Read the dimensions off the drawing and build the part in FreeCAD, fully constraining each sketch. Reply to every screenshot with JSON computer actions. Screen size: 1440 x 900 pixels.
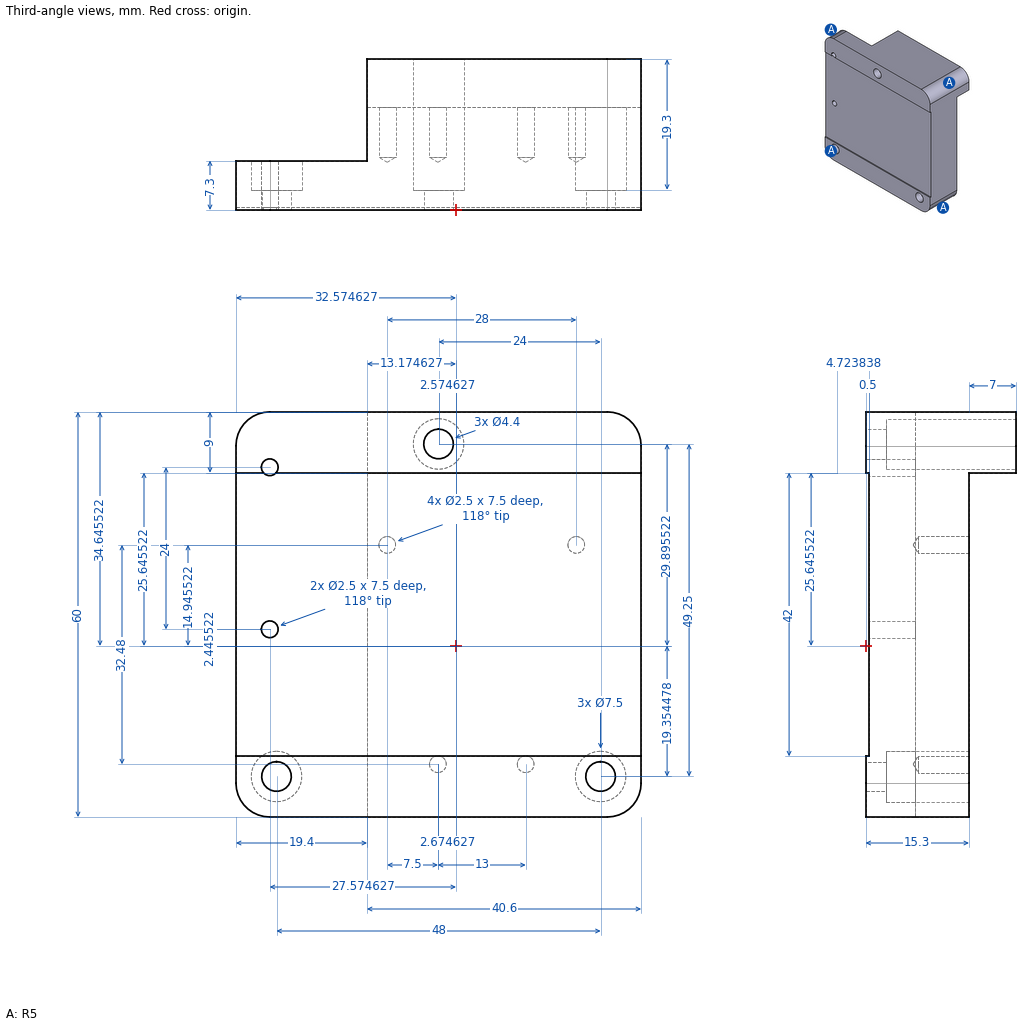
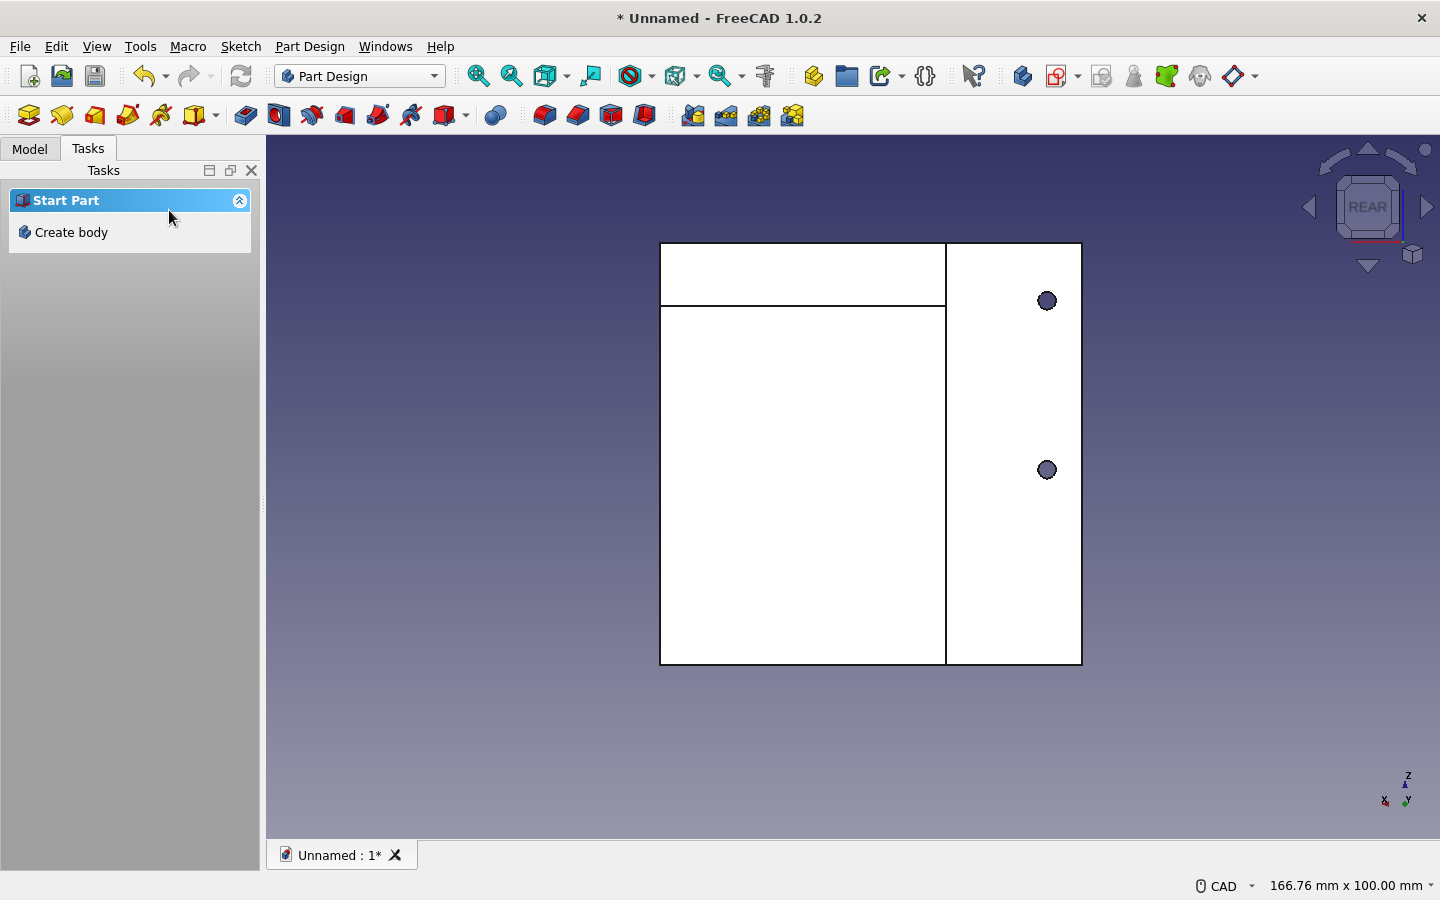
{"action": "left_click", "coordinate": [803, 485]}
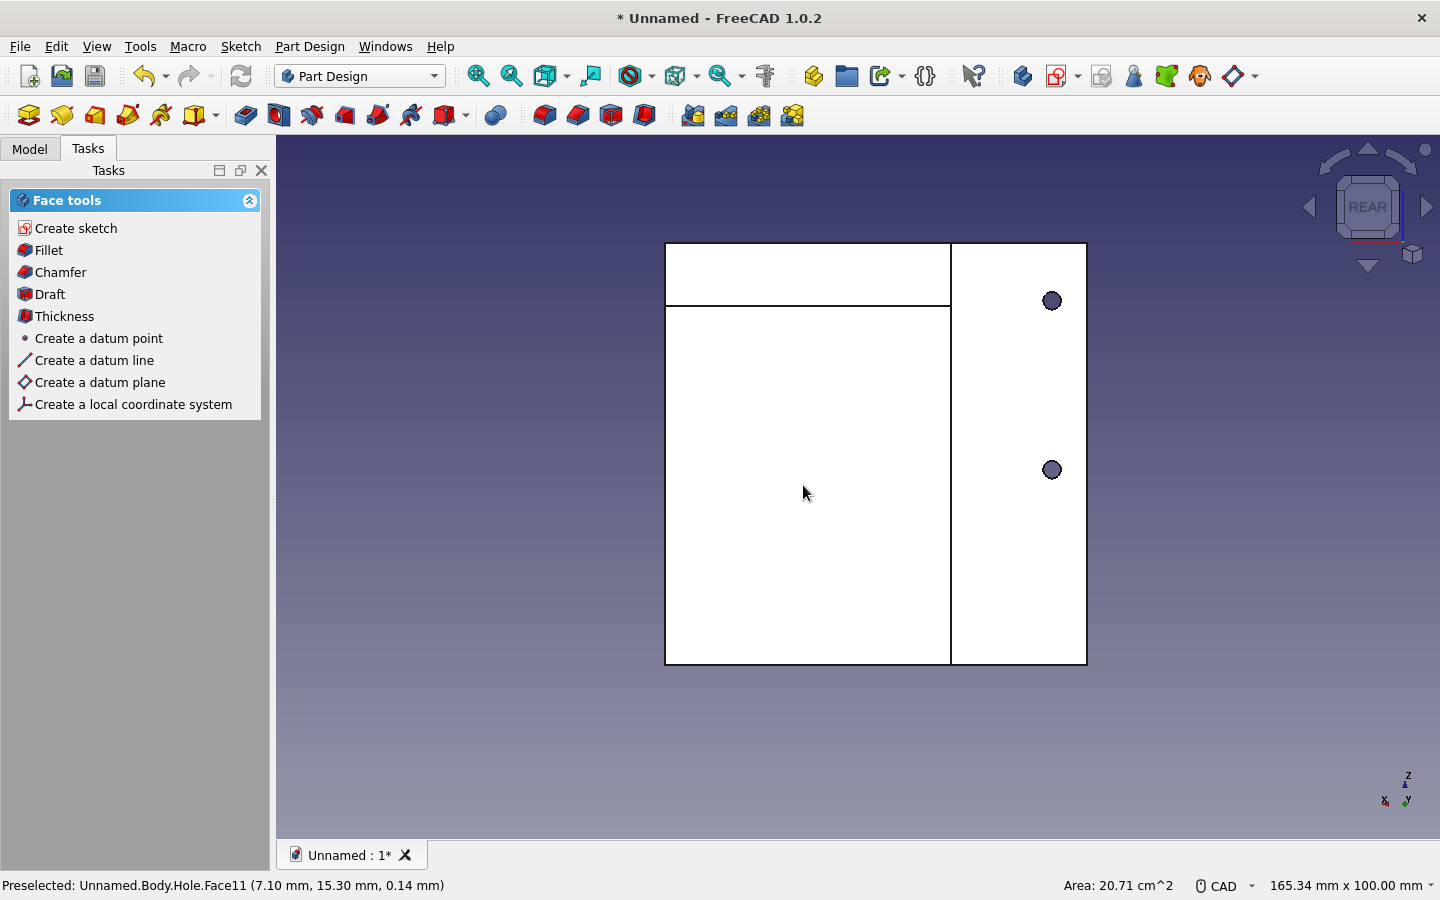
{"action": "left_click", "coordinate": [1056, 76]}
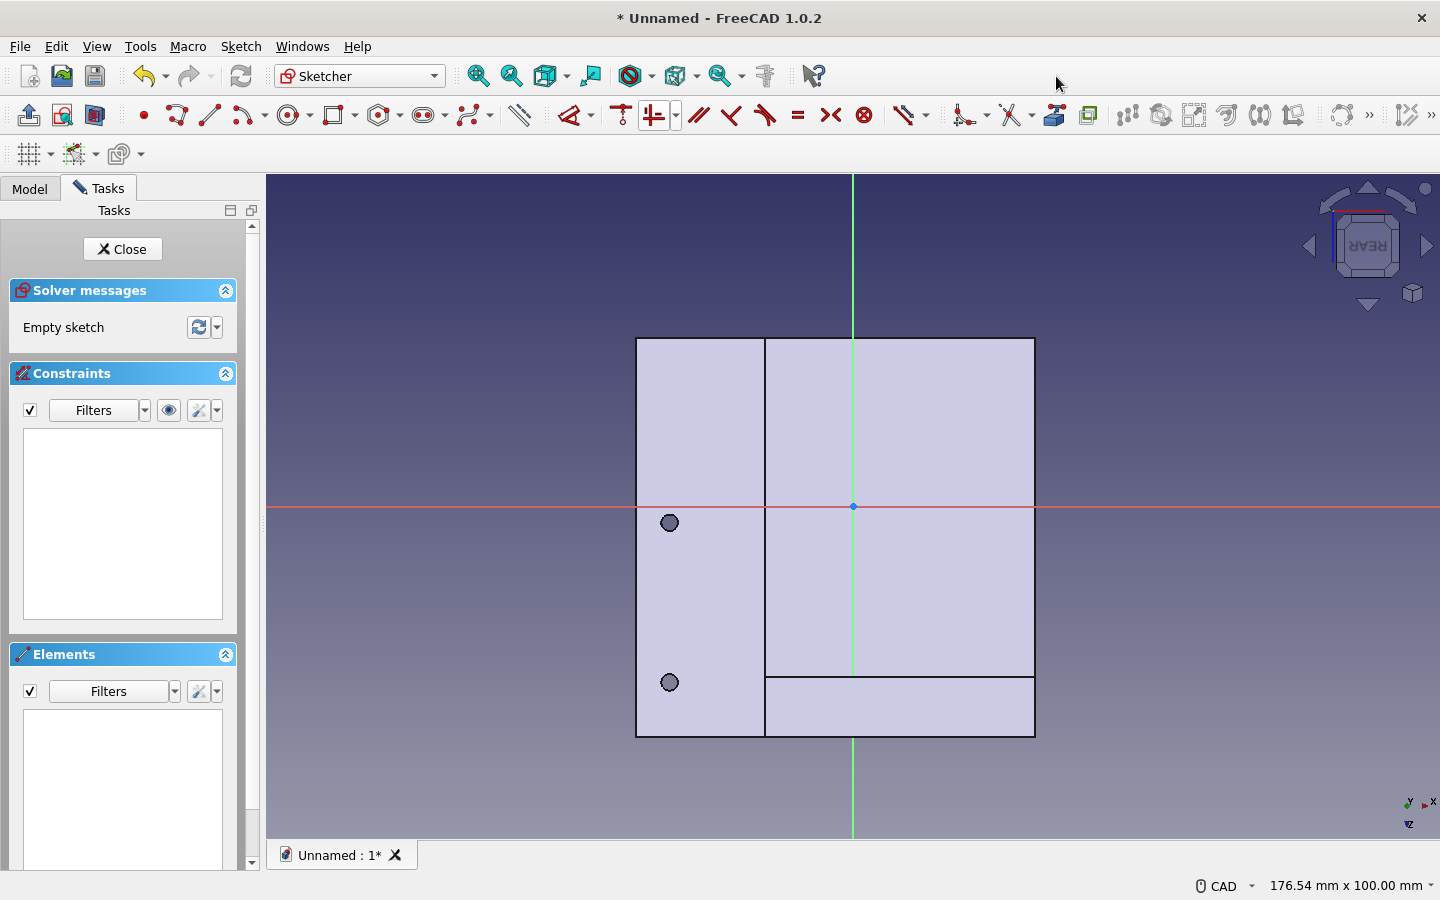
{"action": "scroll", "coordinate": [993, 487], "scroll_direction": "up", "scroll_amount": 3}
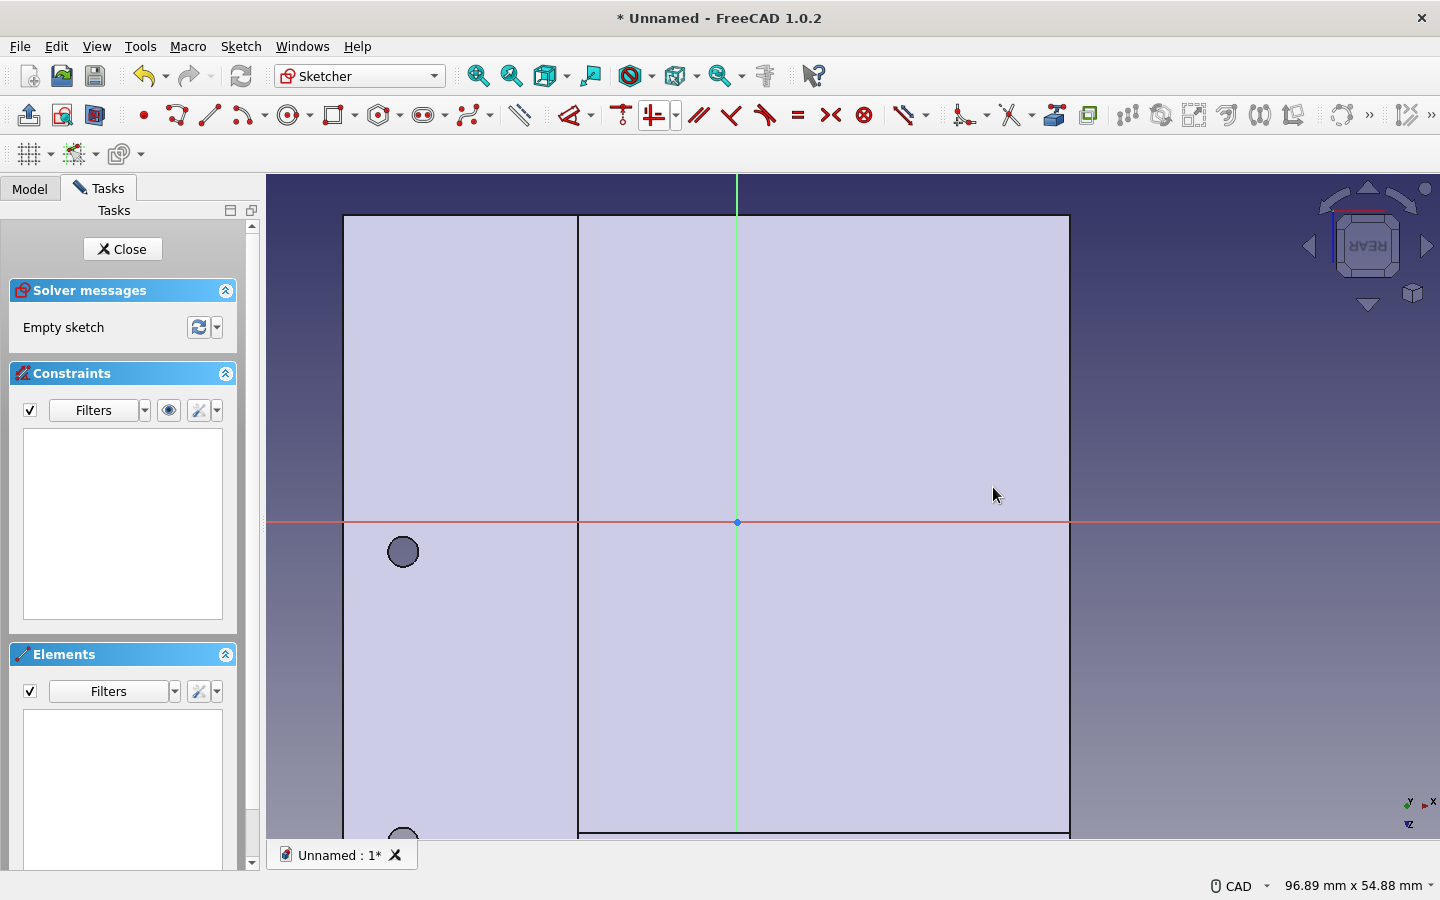
{"action": "key", "text": "g c"}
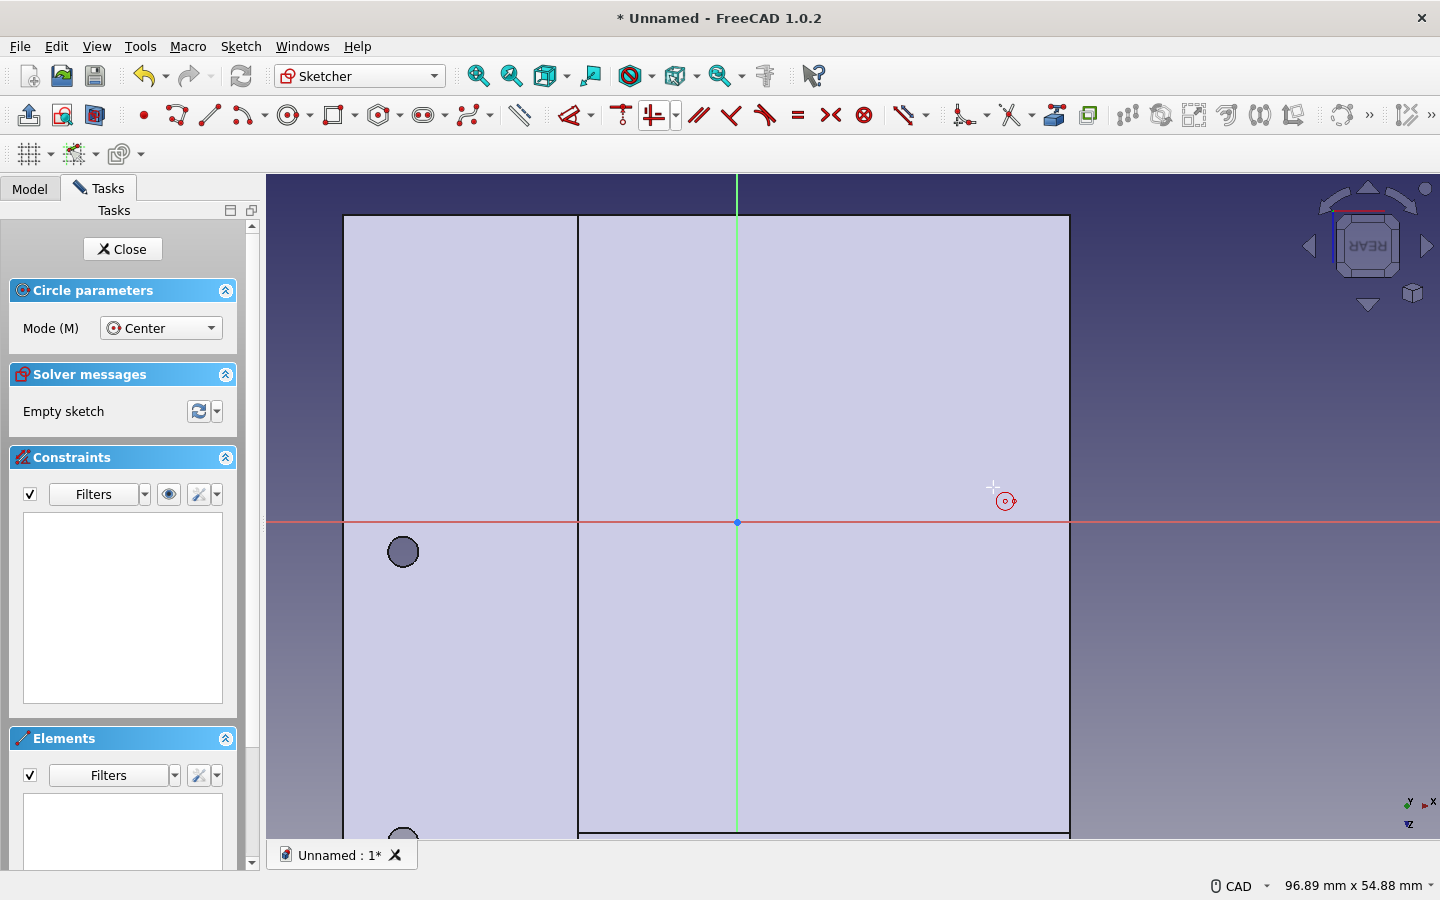
{"action": "scroll", "coordinate": [614, 703], "scroll_direction": "up", "scroll_amount": 3}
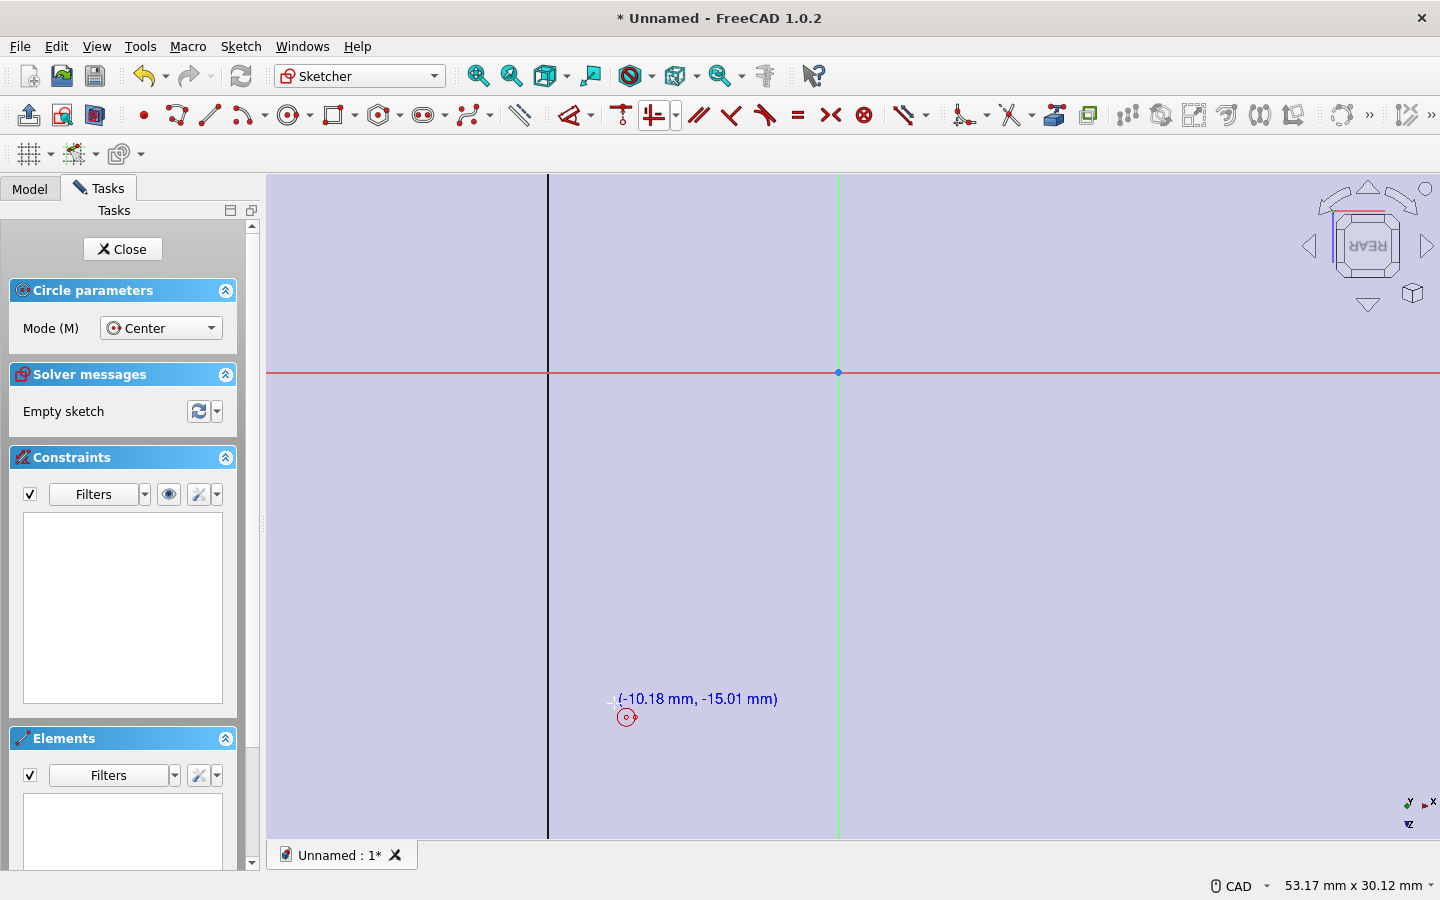
{"action": "left_click", "coordinate": [614, 703]}
{"action": "left_click", "coordinate": [633, 683]}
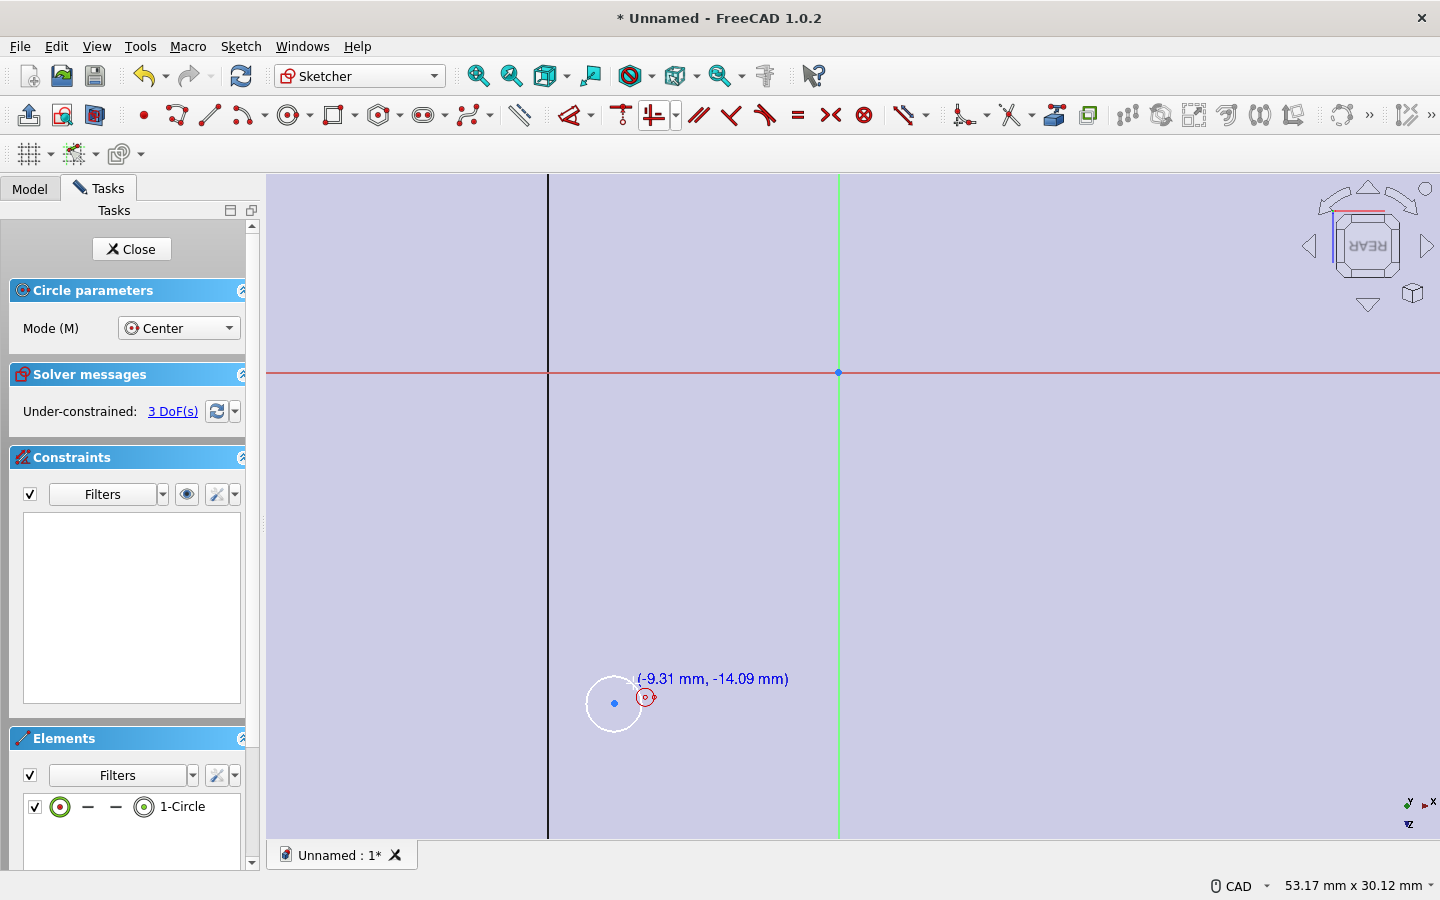
{"action": "left_click", "coordinate": [1232, 703]}
{"action": "left_click", "coordinate": [1252, 683]}